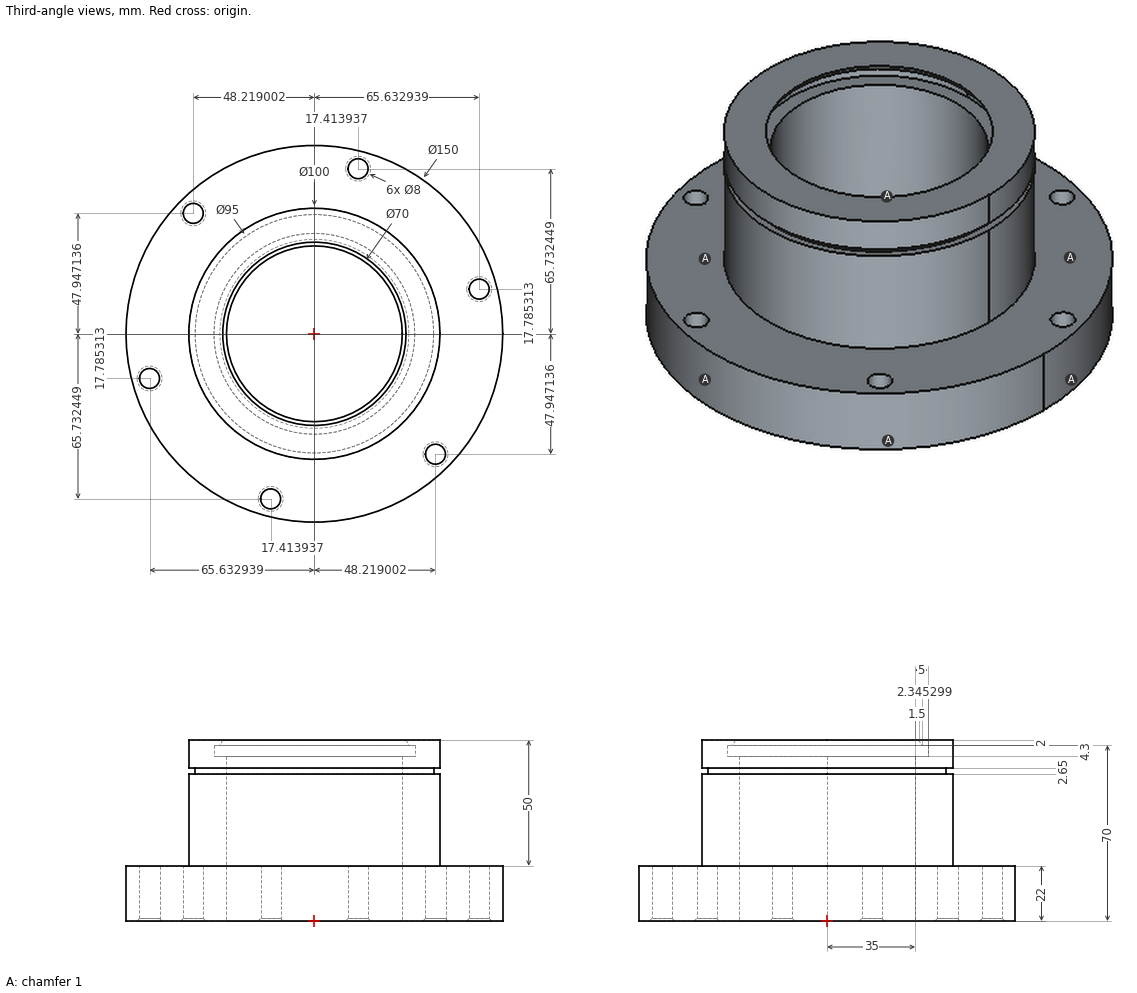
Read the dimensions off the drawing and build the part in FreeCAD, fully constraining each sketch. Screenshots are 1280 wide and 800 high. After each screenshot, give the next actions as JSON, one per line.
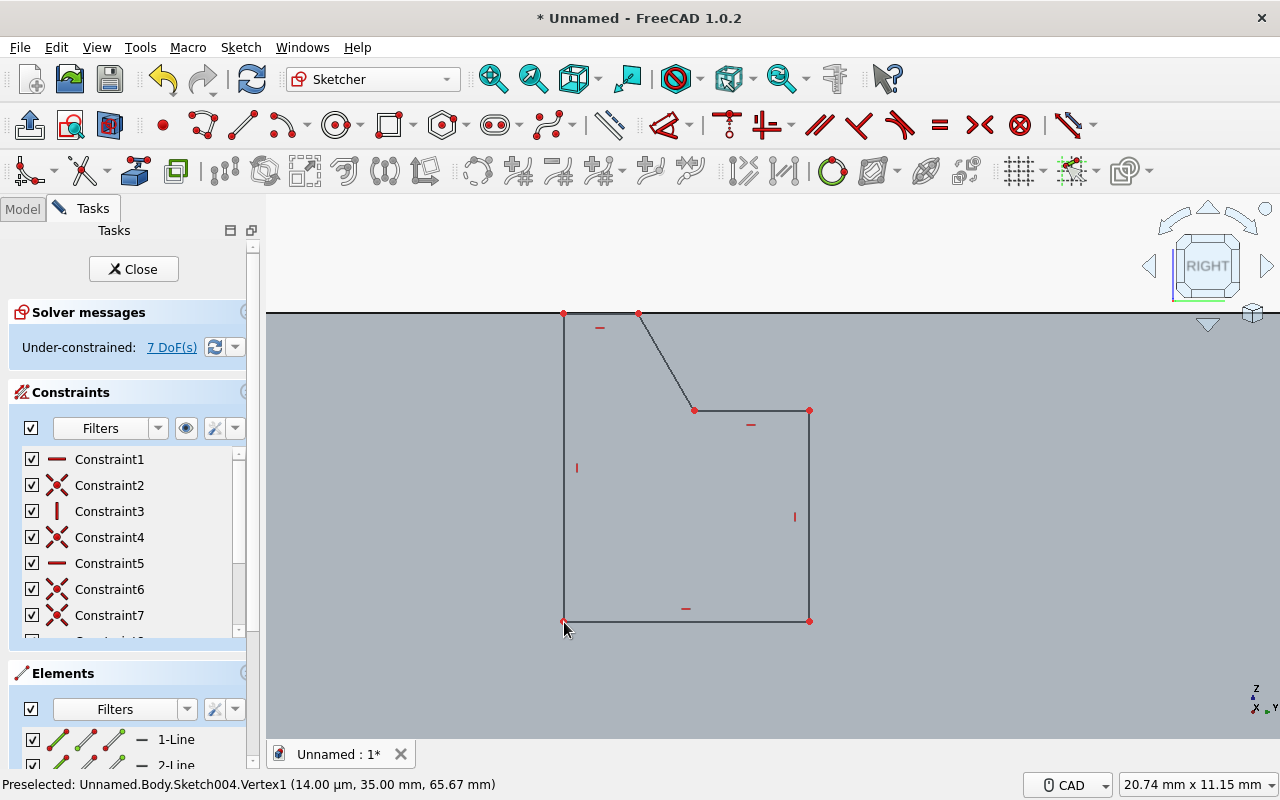
{"action": "left_click", "coordinate": [664, 126]}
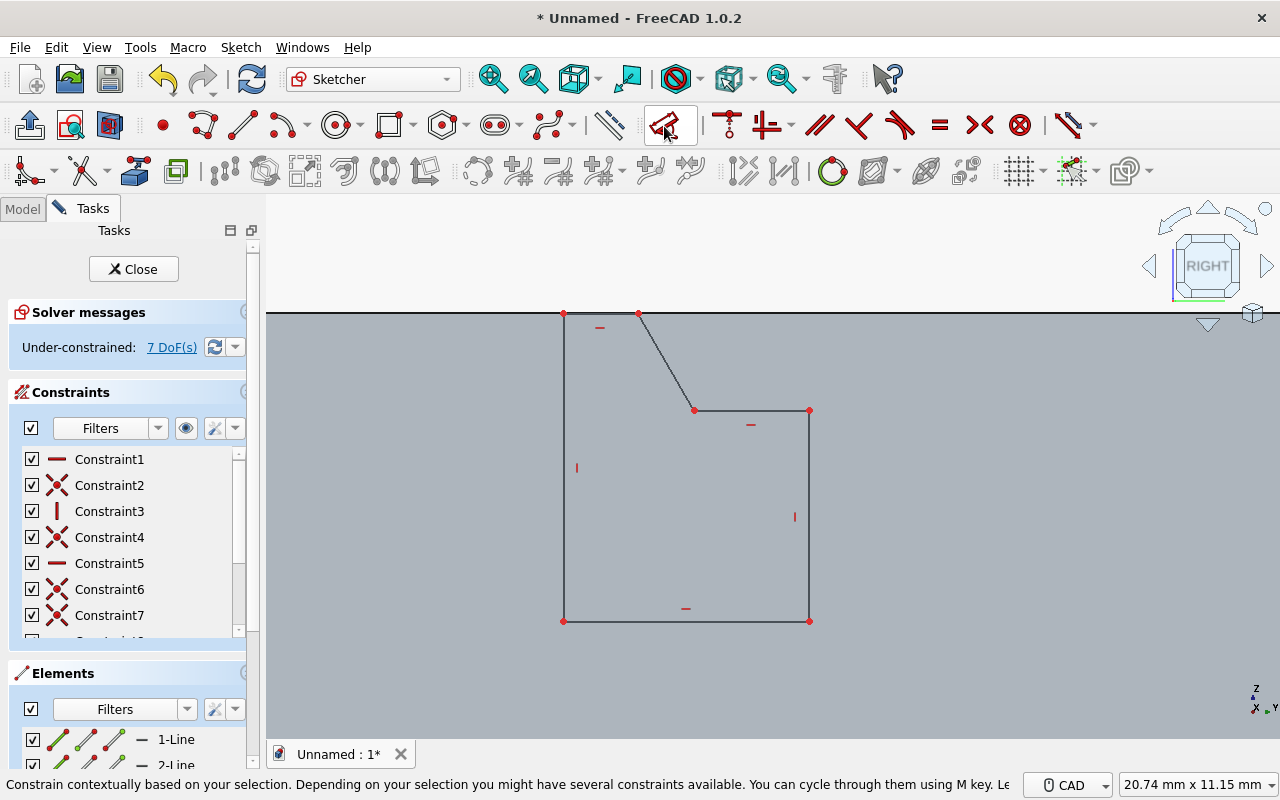
{"action": "left_click", "coordinate": [637, 622]}
{"action": "left_click", "coordinate": [686, 656]}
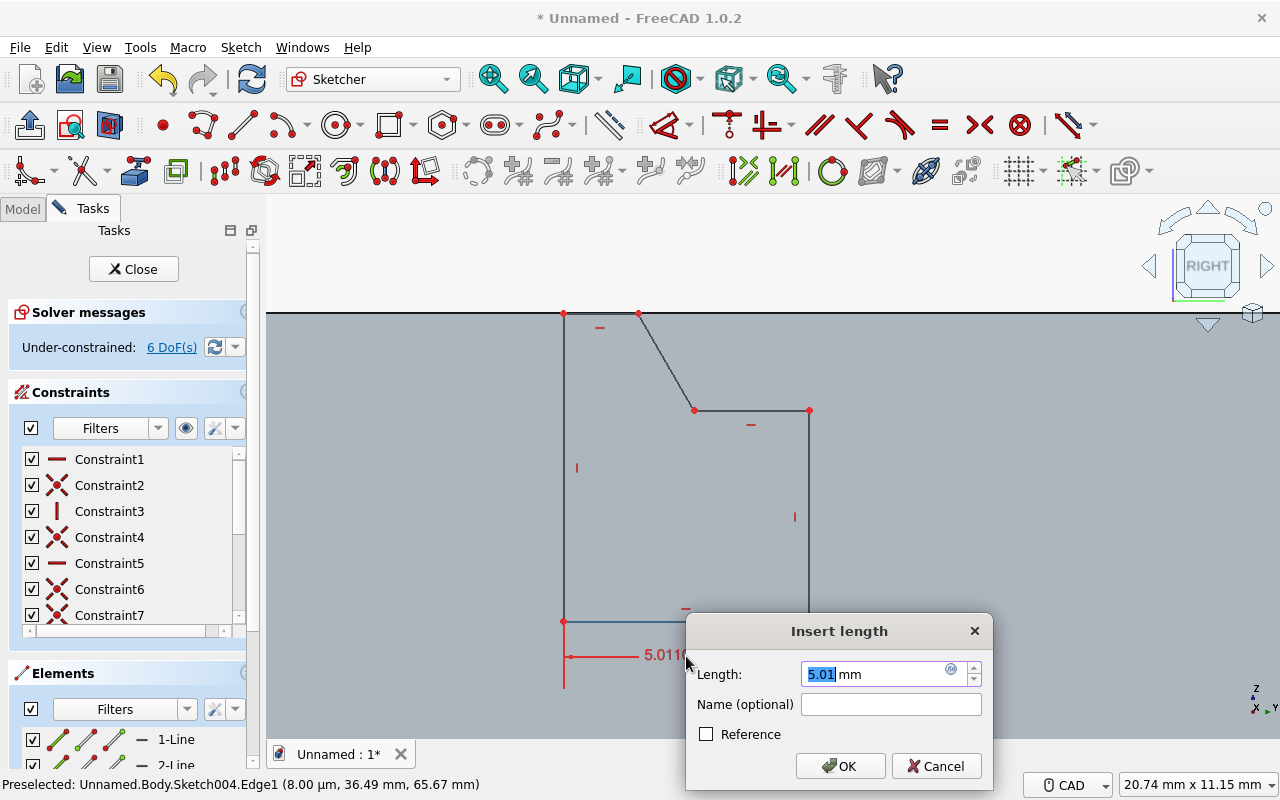
{"action": "type", "text": "5"}
{"action": "key", "text": "Return"}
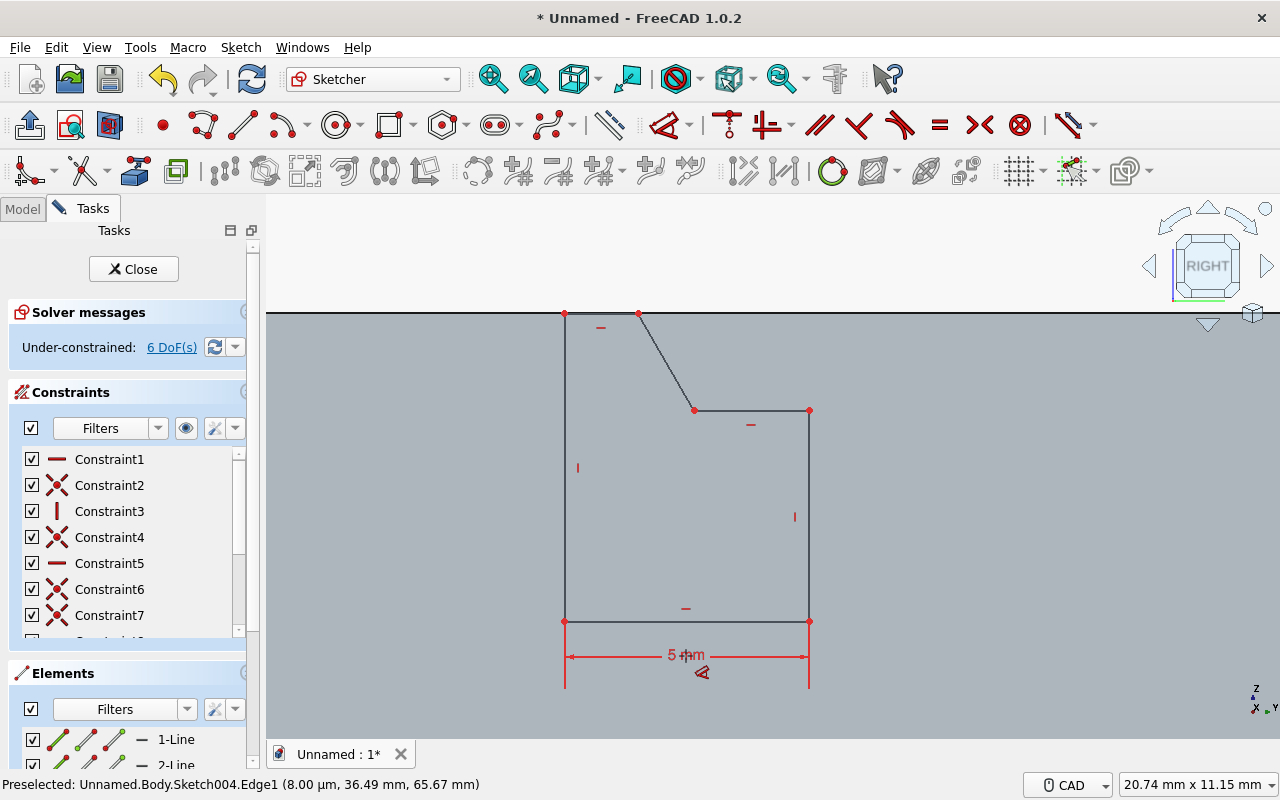
{"action": "left_click", "coordinate": [677, 382]}
{"action": "left_click", "coordinate": [604, 362]}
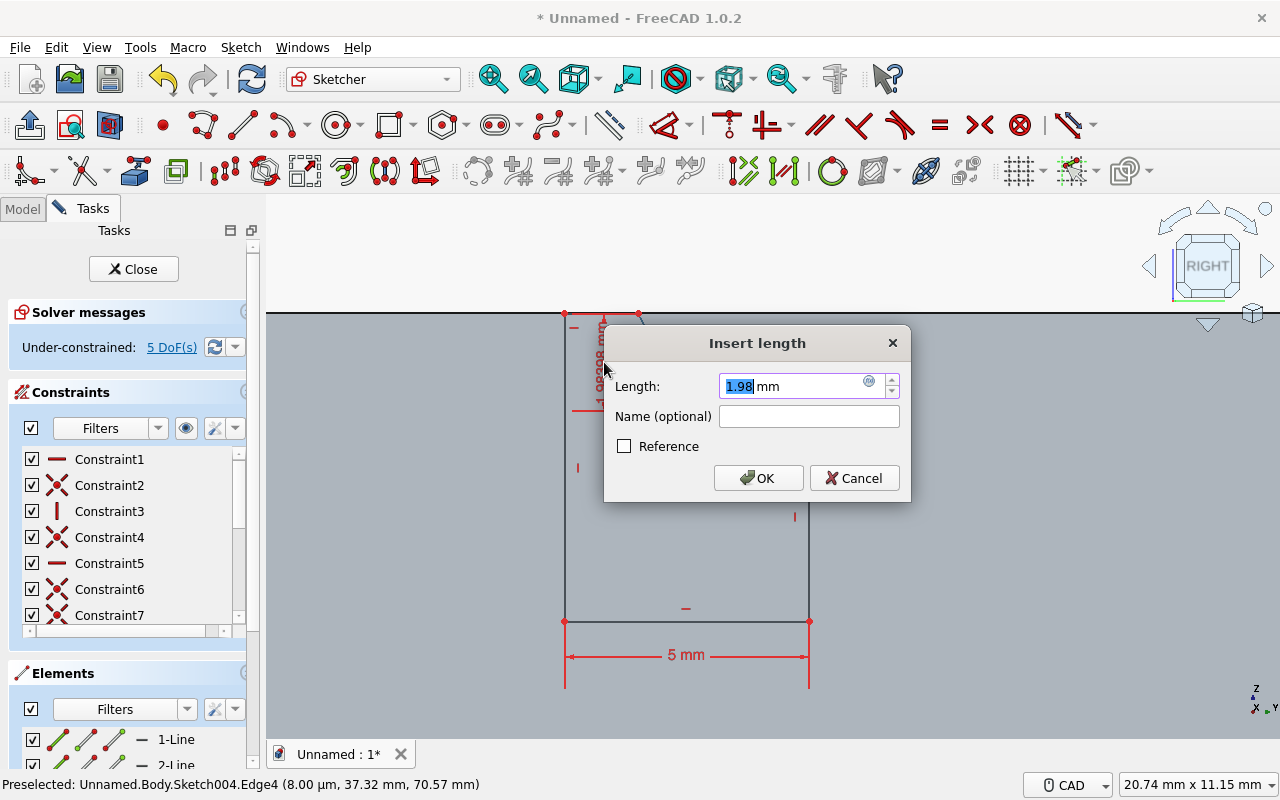
{"action": "type", "text": "2"}
{"action": "key", "text": "Return"}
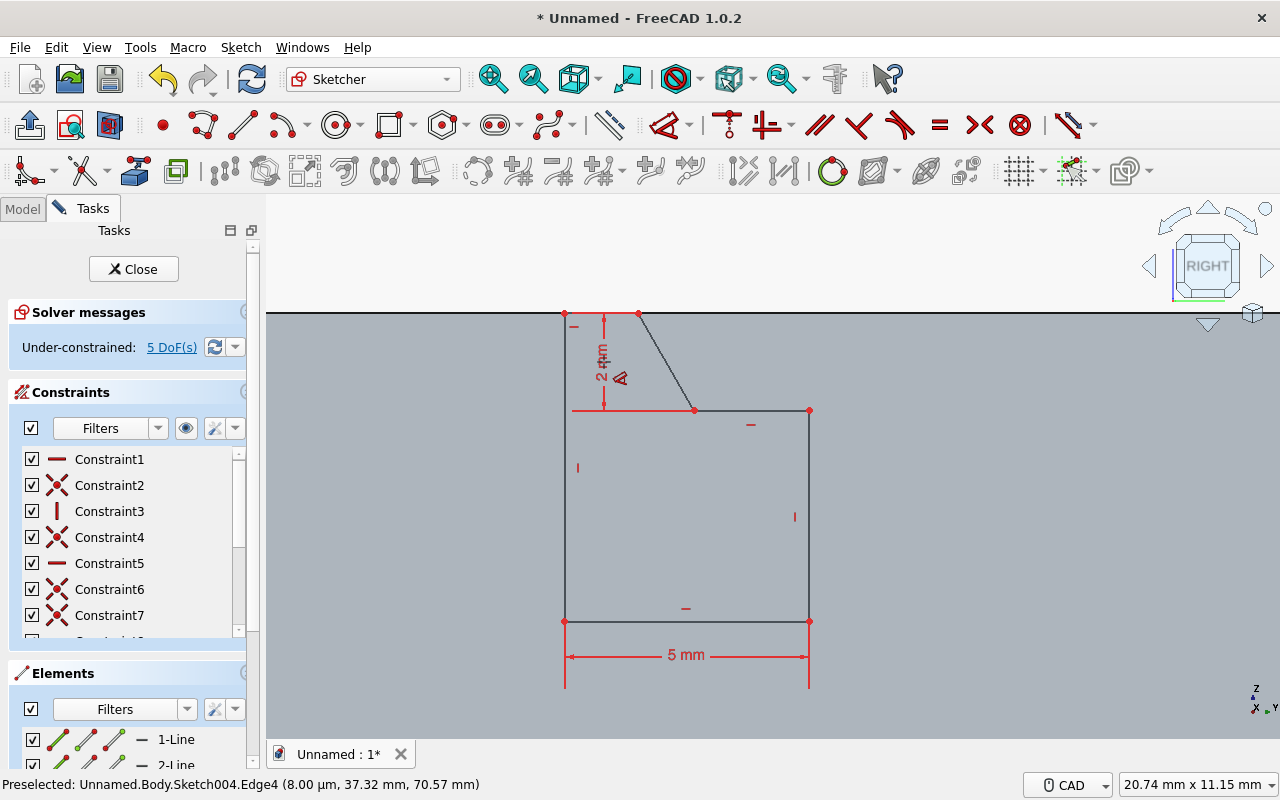
{"action": "left_click", "coordinate": [809, 559]}
{"action": "left_click", "coordinate": [843, 516]}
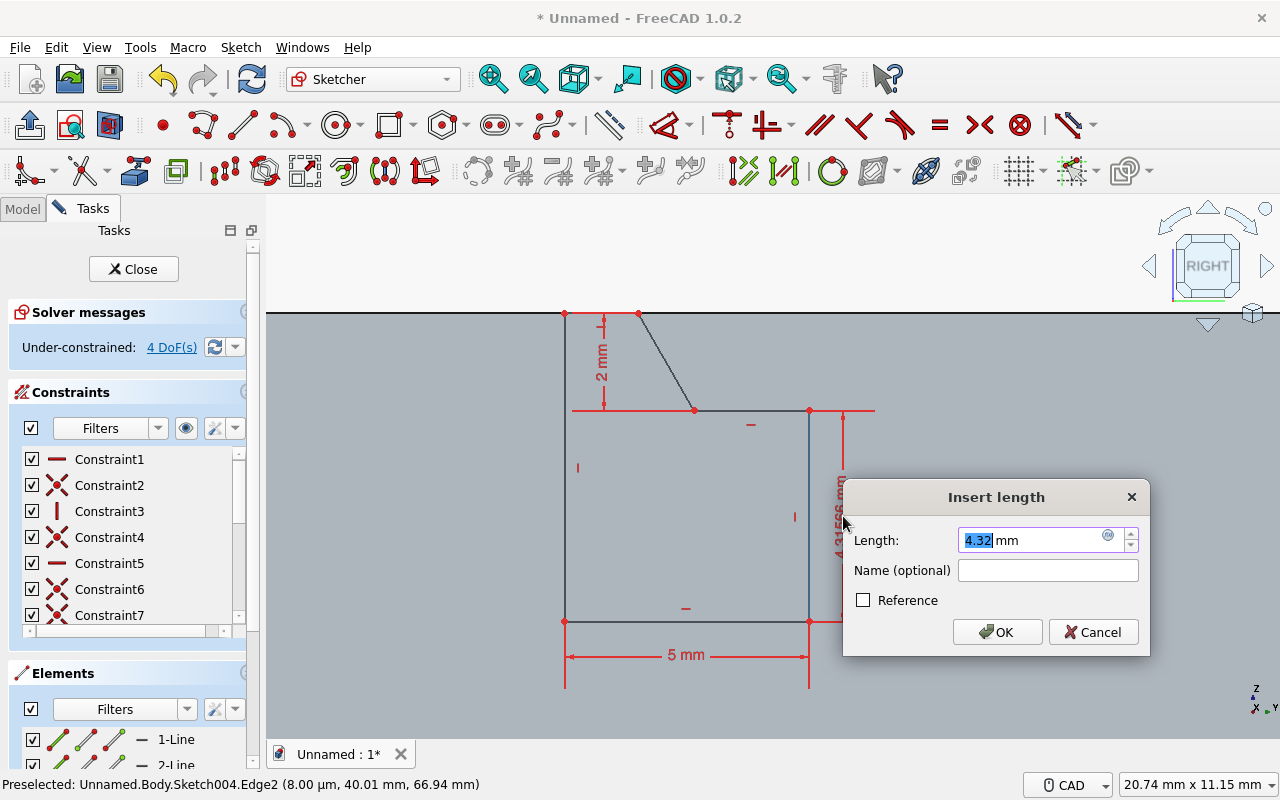
{"action": "type", "text": "4.3"}
{"action": "key", "text": "Return"}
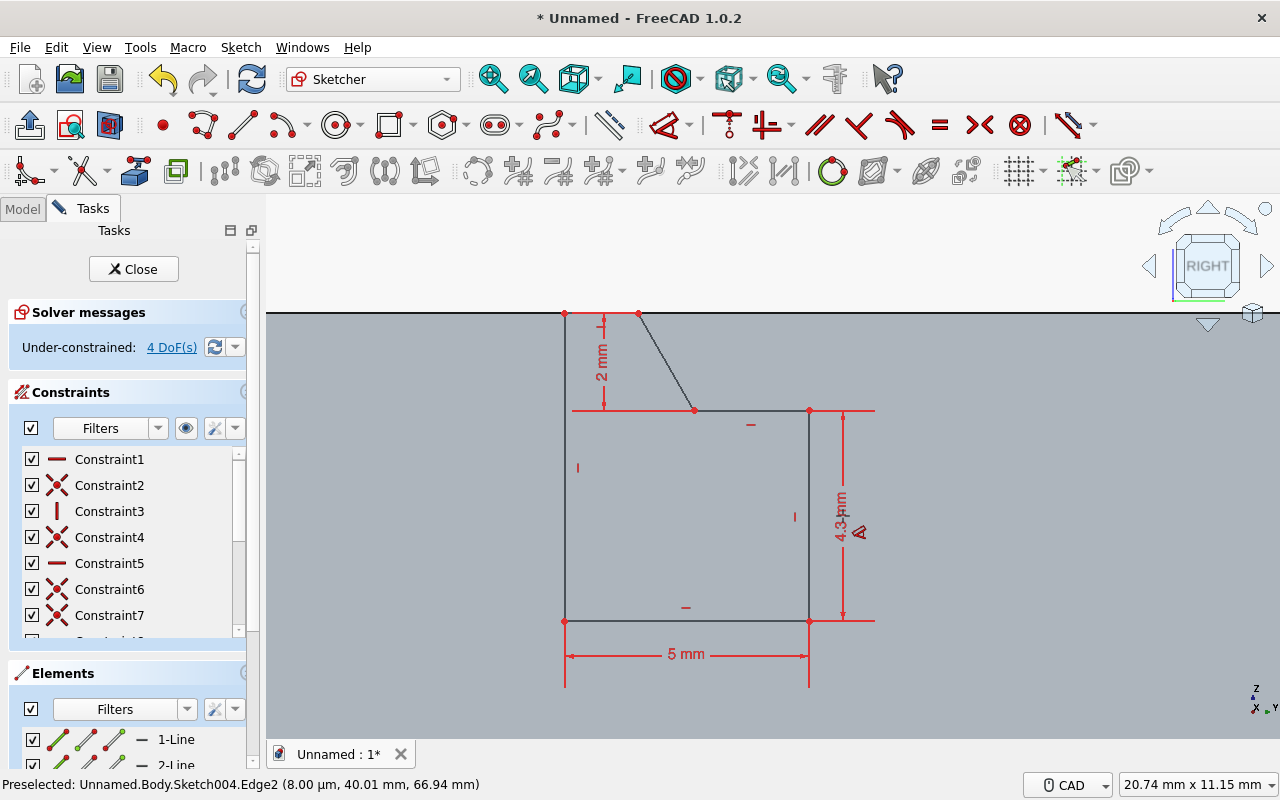
{"action": "left_click", "coordinate": [616, 313]}
{"action": "left_click", "coordinate": [601, 279]}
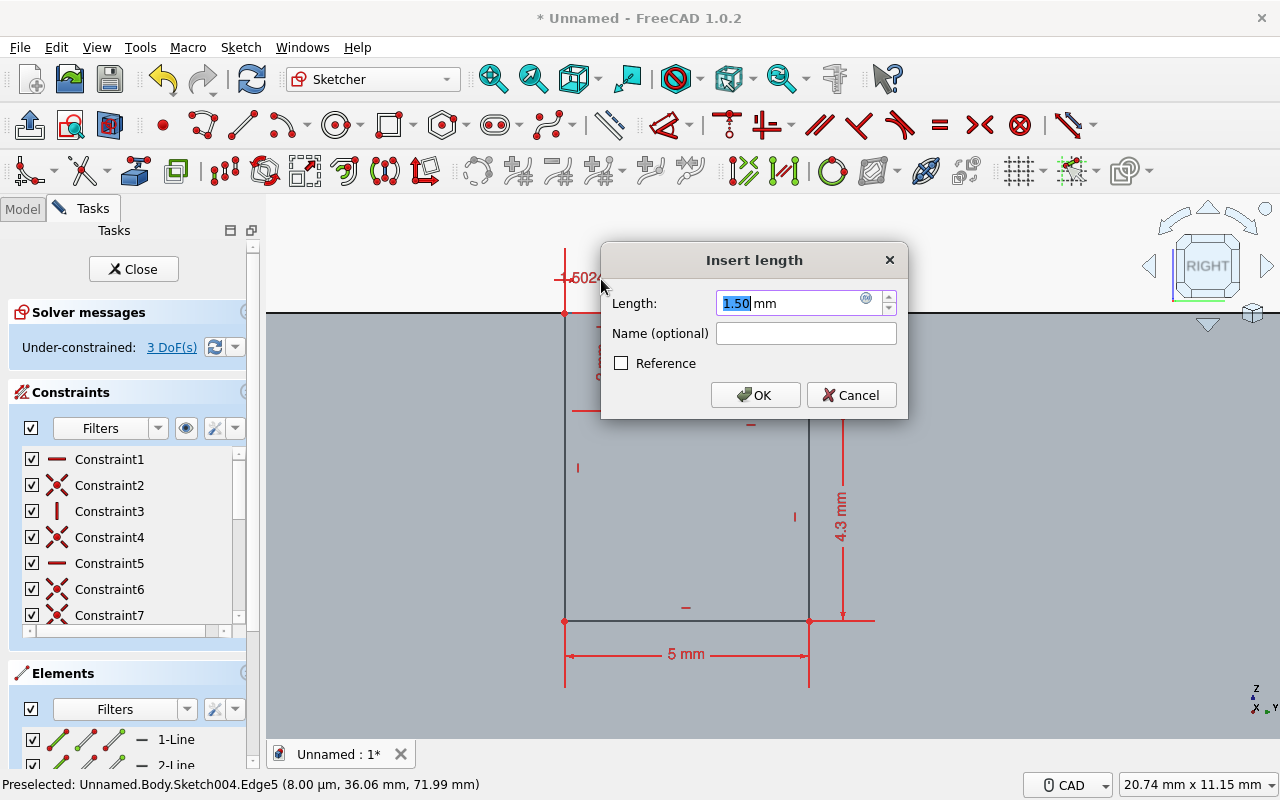
{"action": "type", "text": "1.5"}
{"action": "key", "text": "Return"}